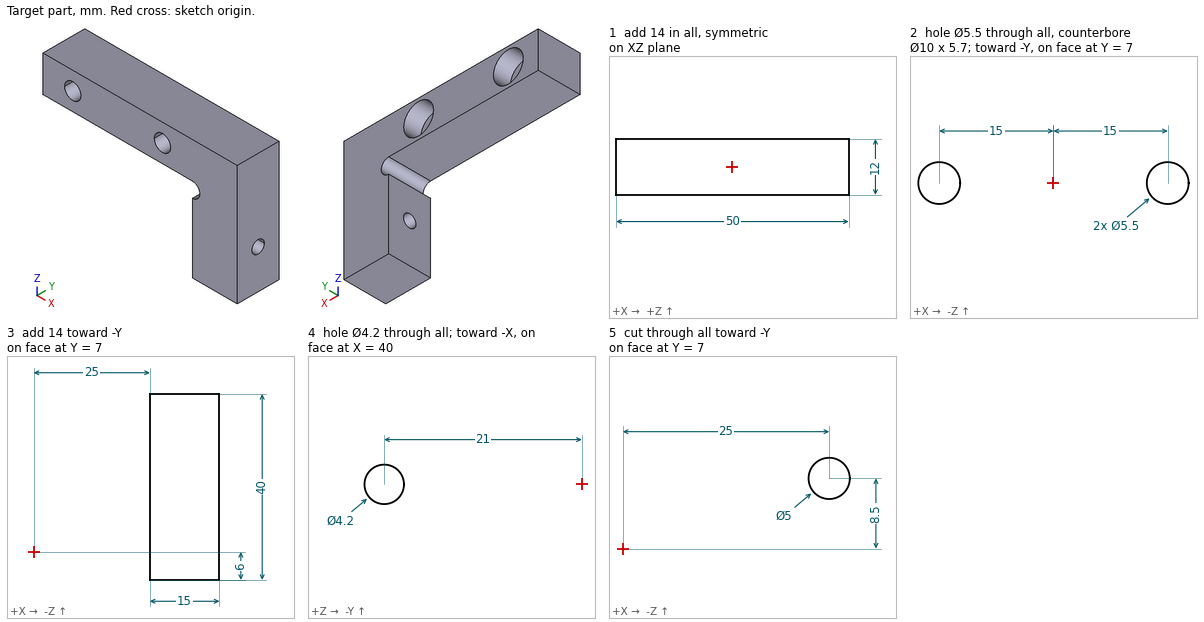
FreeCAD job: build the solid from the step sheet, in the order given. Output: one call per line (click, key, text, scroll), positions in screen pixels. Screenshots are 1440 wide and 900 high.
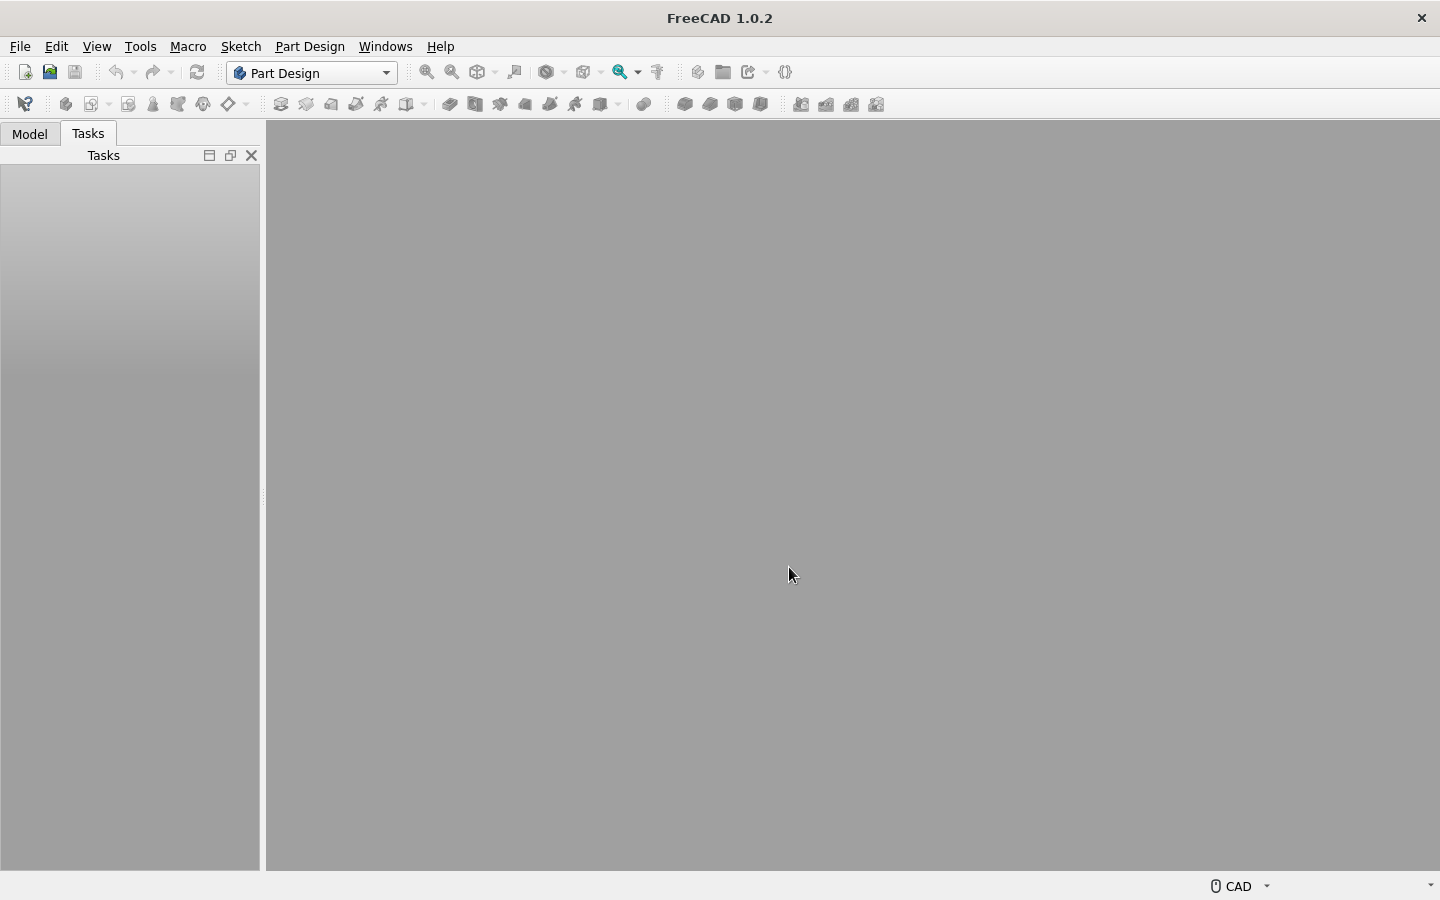
key(ctrl+n)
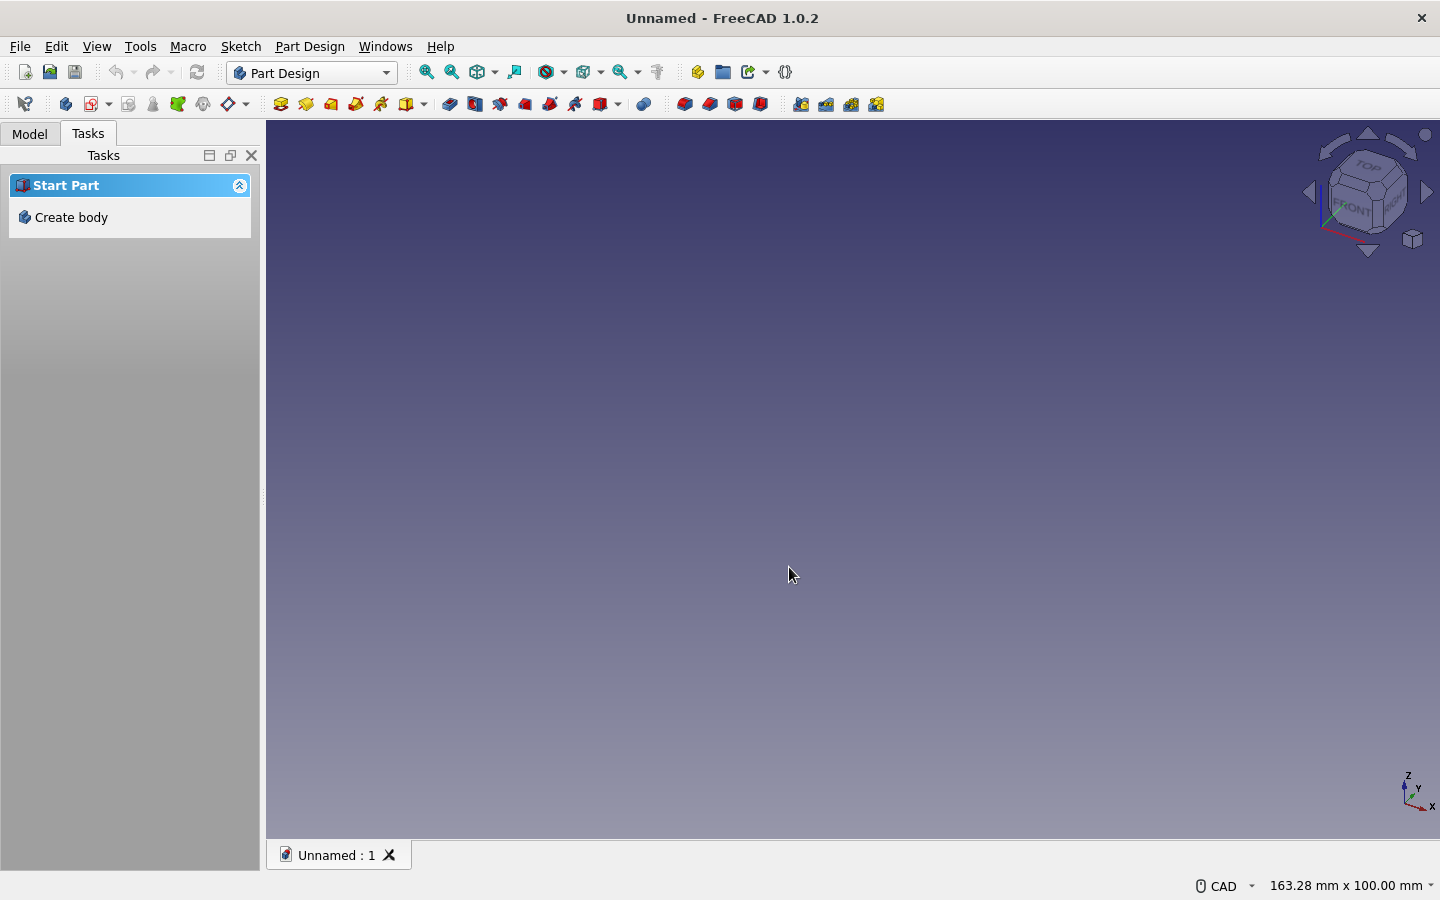
click(90, 104)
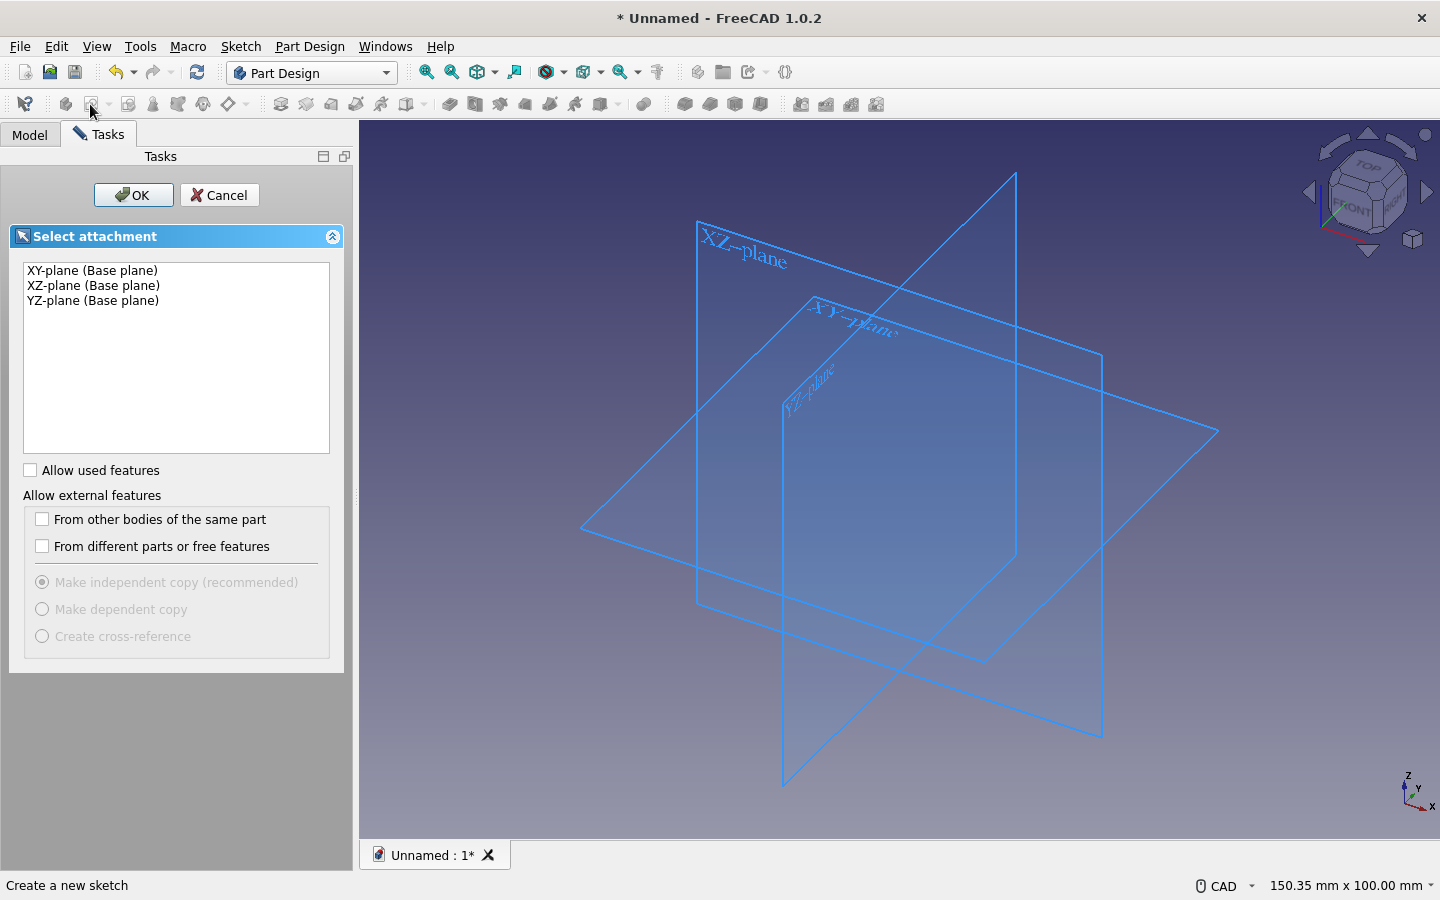
click(84, 286)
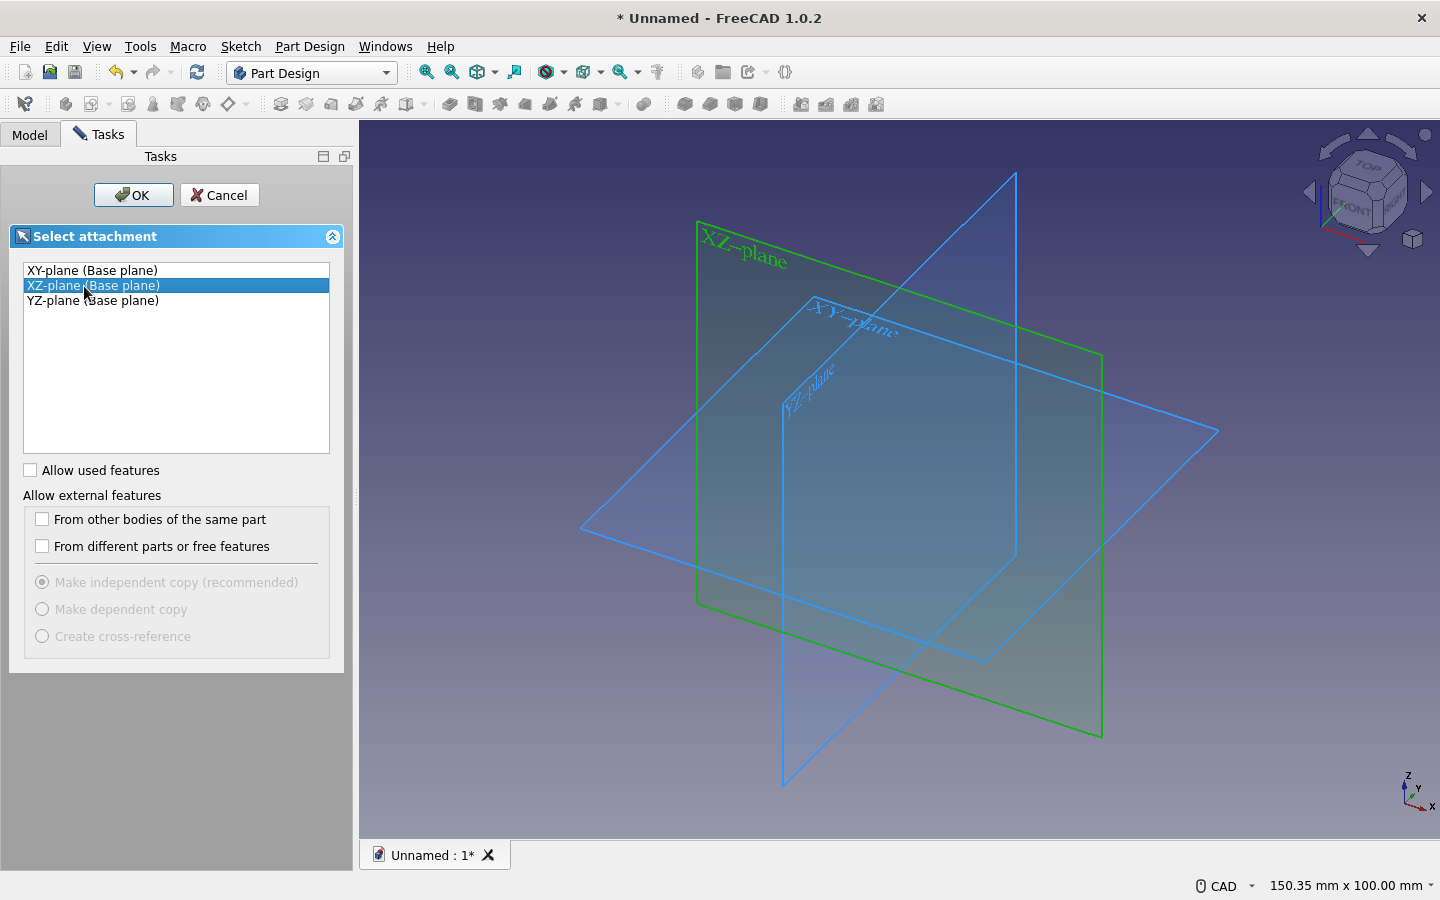
click(134, 195)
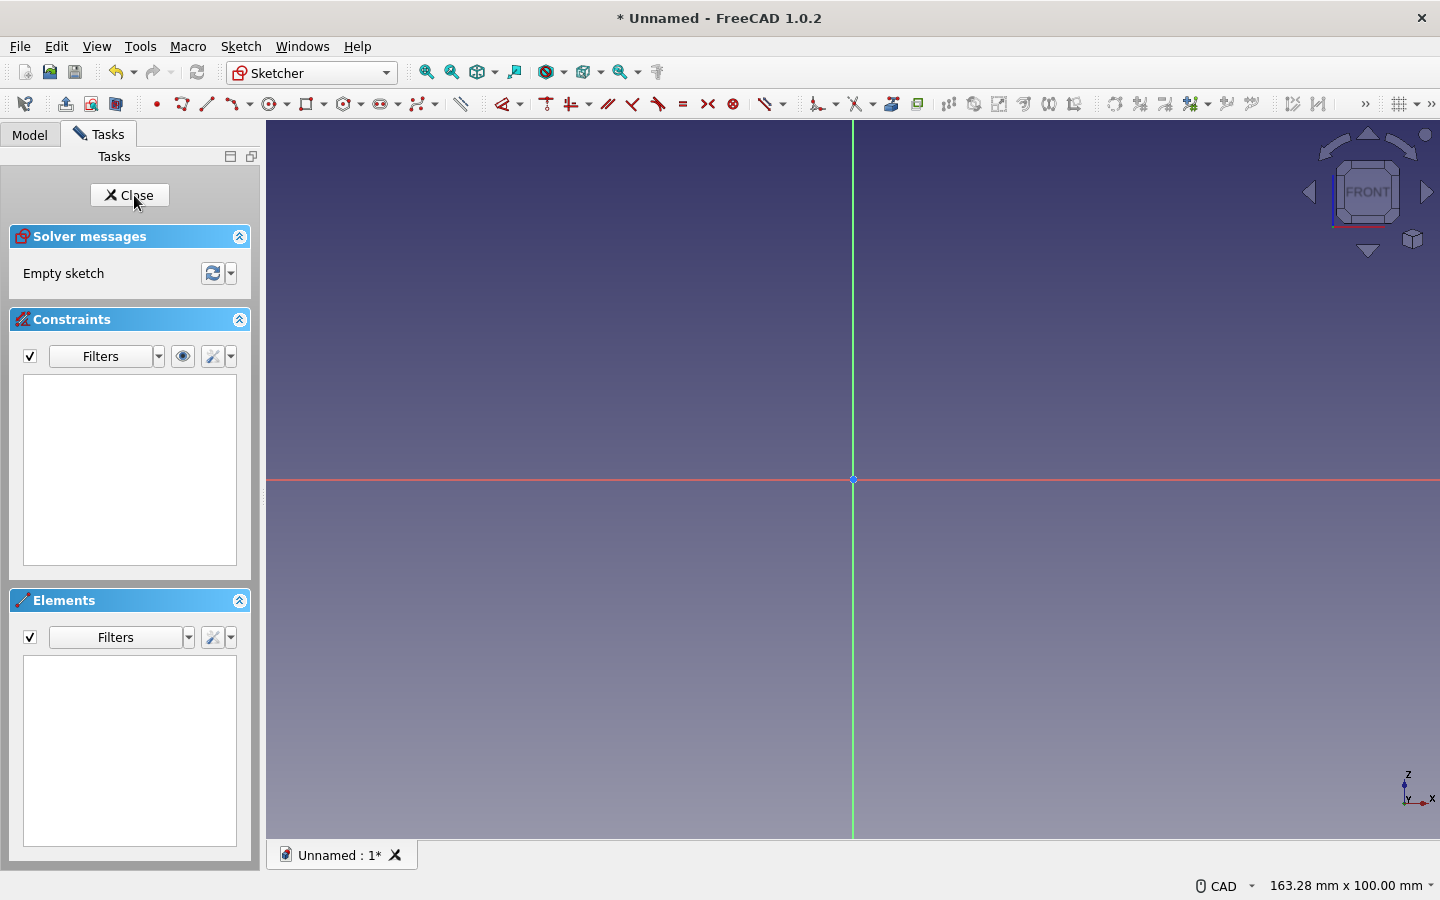
scroll(936, 480, up, 3)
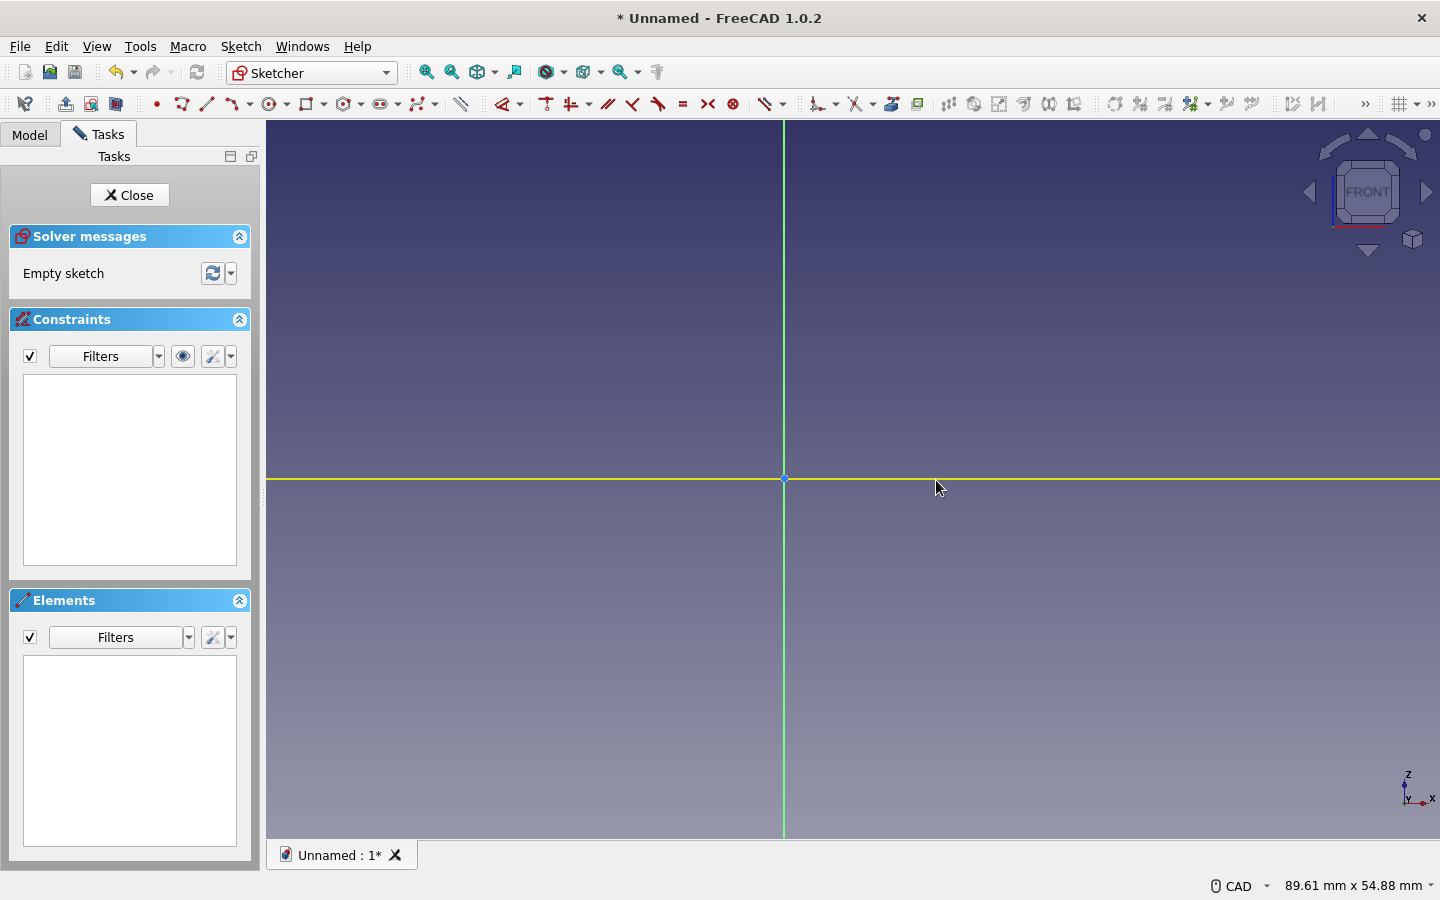
key(g)
key(v)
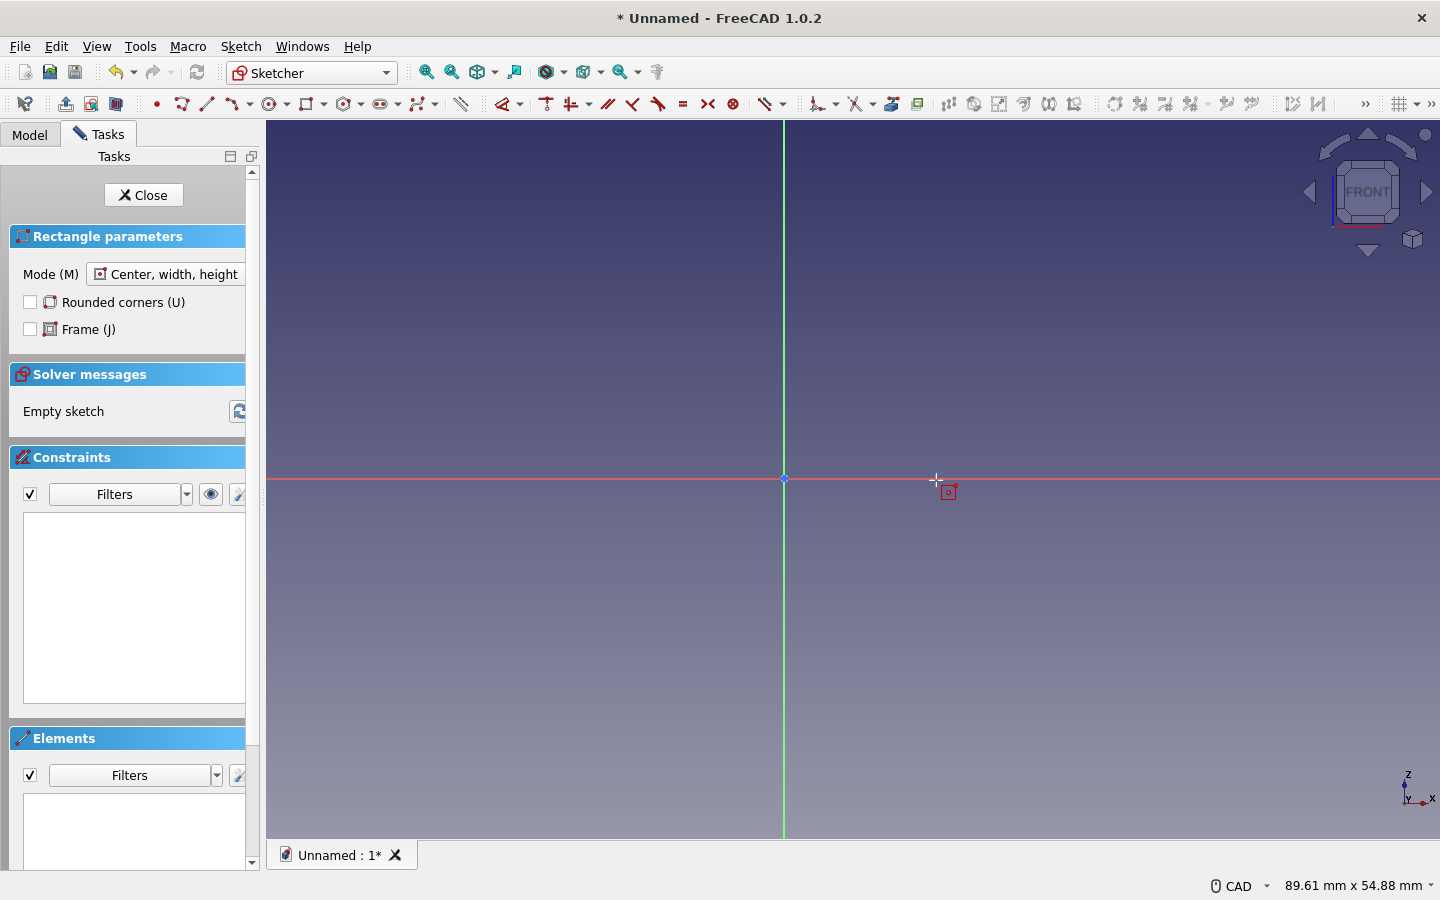
click(784, 479)
move(1112, 400)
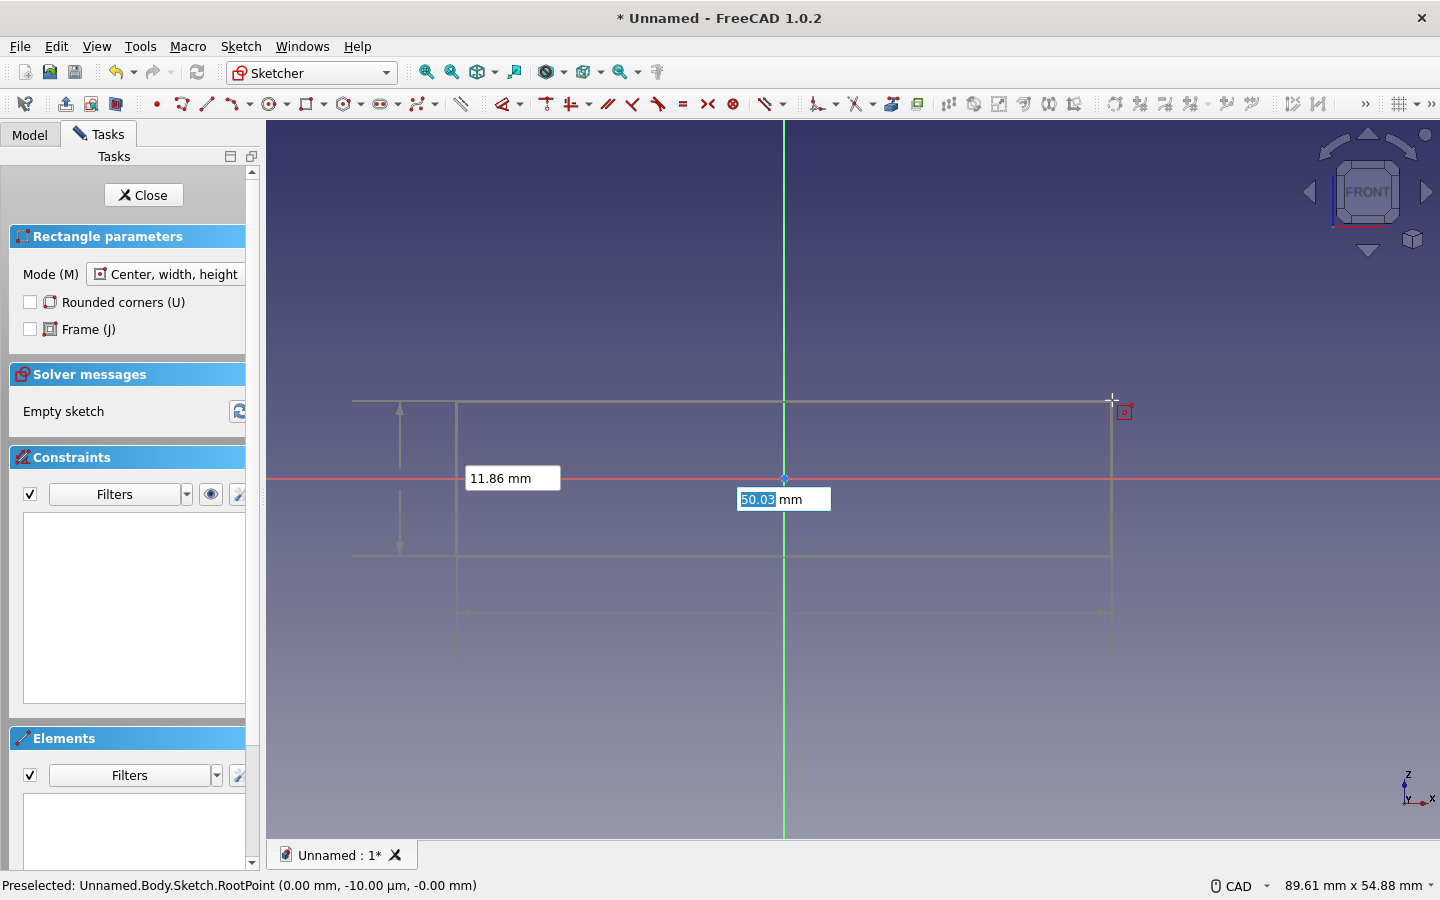
text(50)
key(Tab)
text(12)
key(Return)
key(Escape)